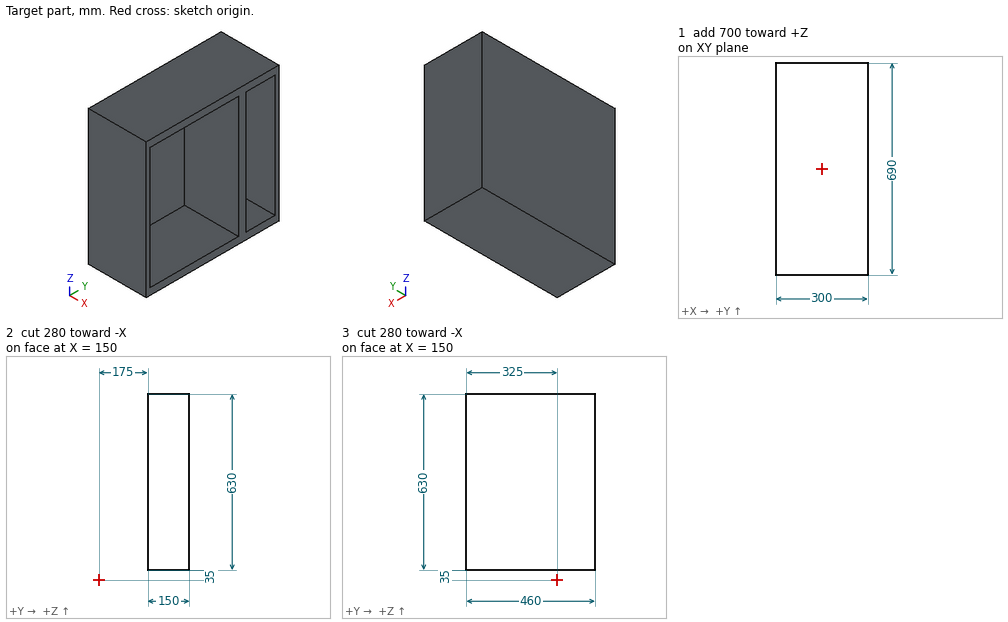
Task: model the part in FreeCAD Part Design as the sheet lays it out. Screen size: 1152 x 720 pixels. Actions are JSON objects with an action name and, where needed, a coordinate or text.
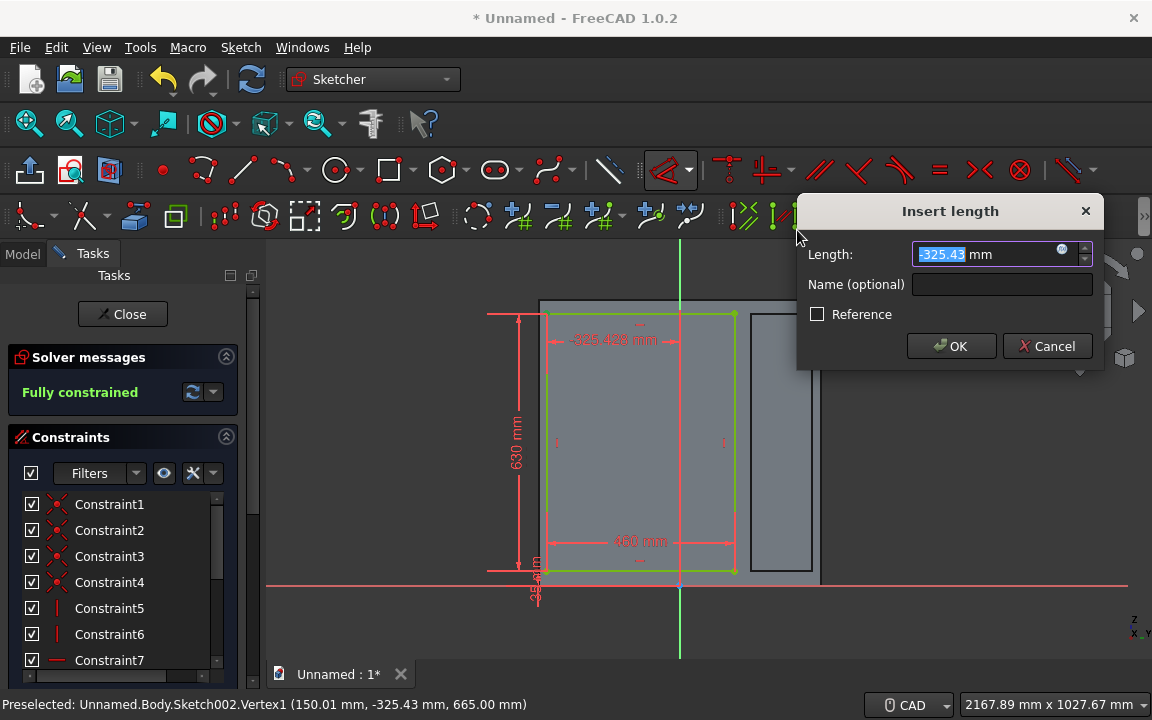
{"action": "type", "text": "-325"}
{"action": "key", "text": "Return"}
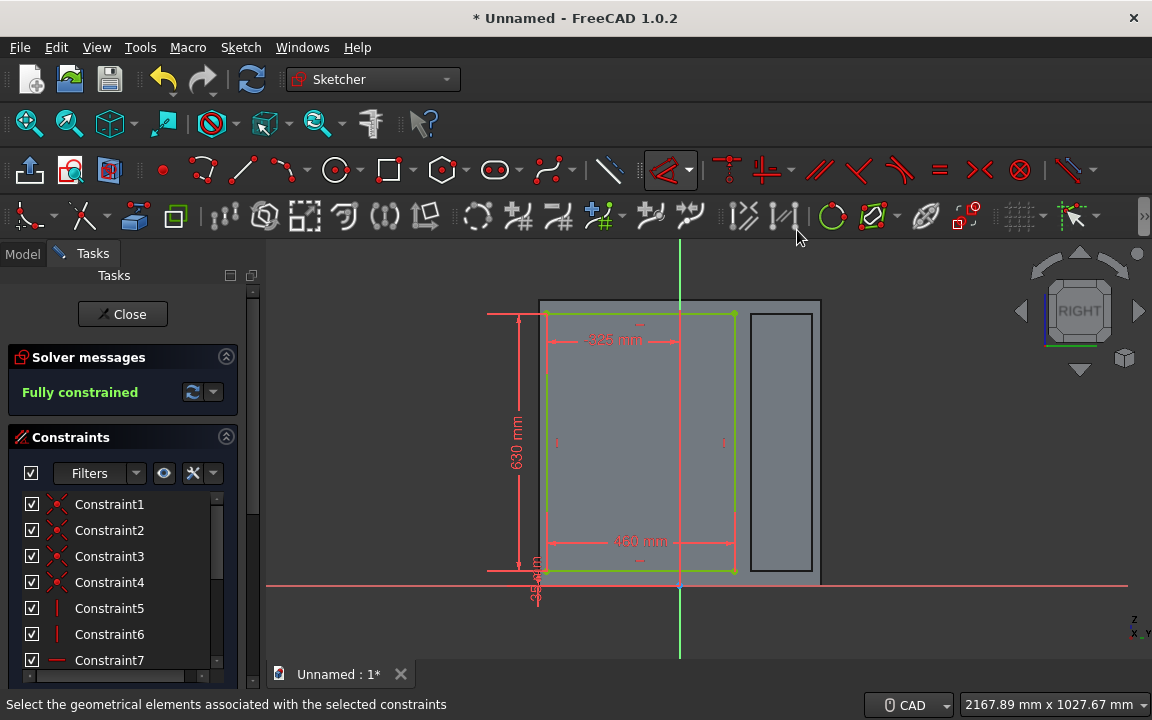
{"action": "left_click", "coordinate": [123, 314]}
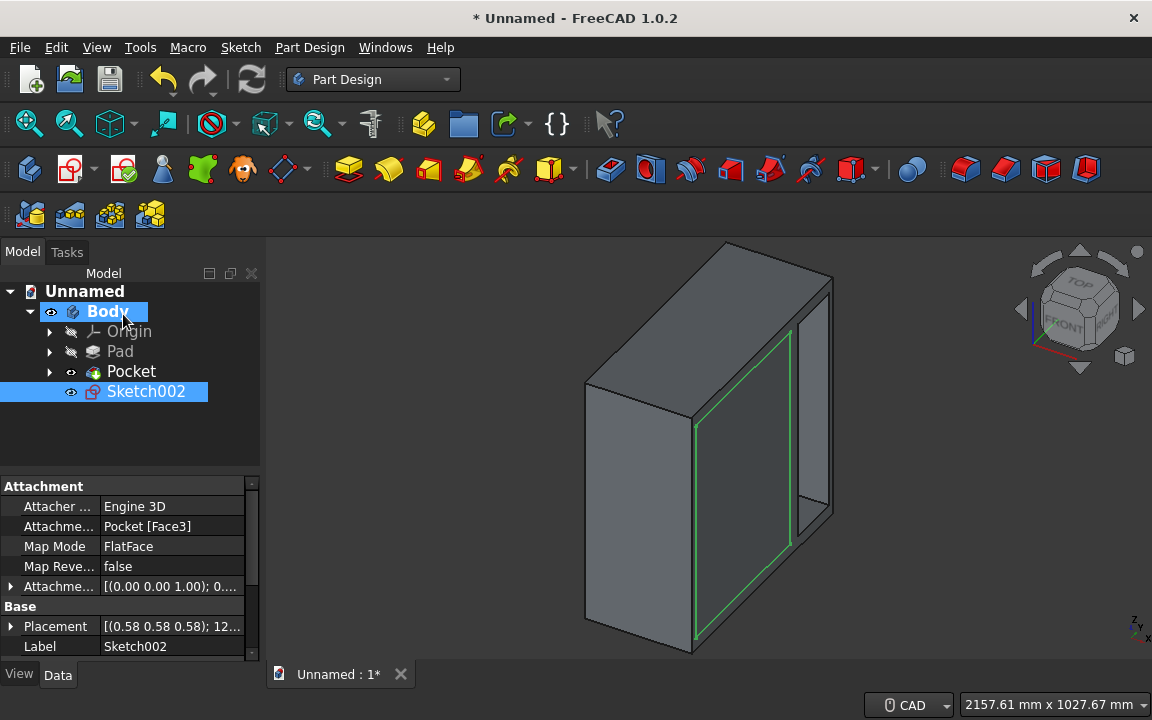
{"action": "left_click", "coordinate": [612, 170]}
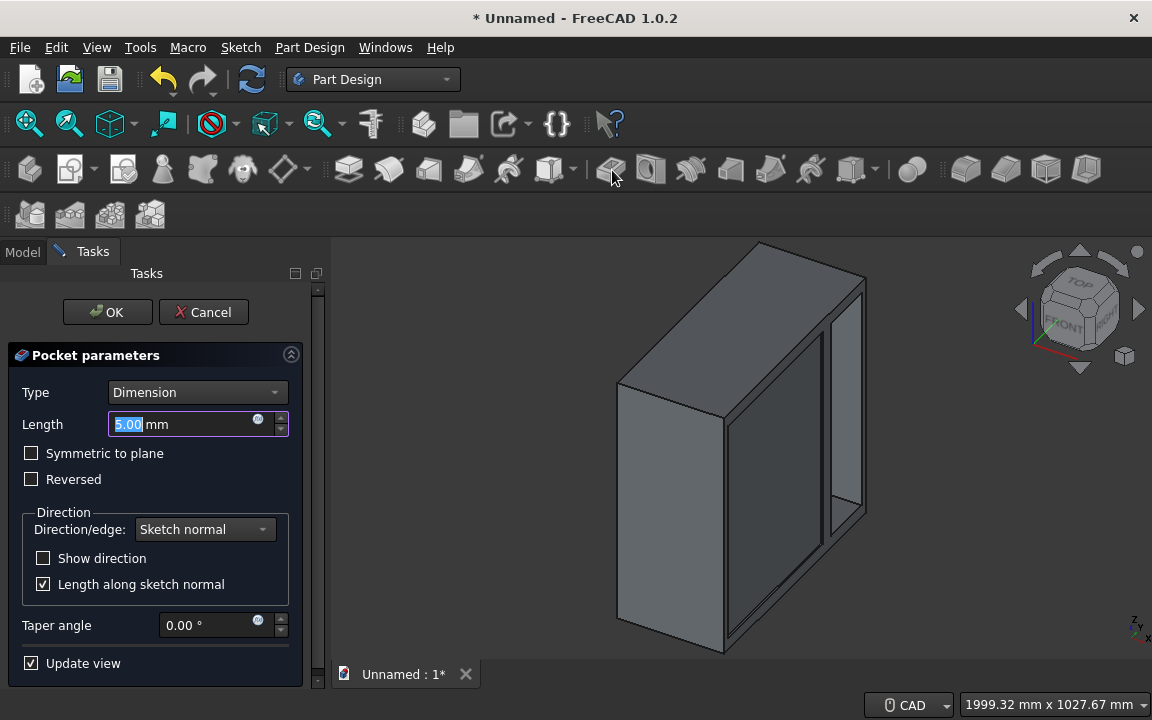
{"action": "type", "text": "280"}
{"action": "key", "text": "Tab"}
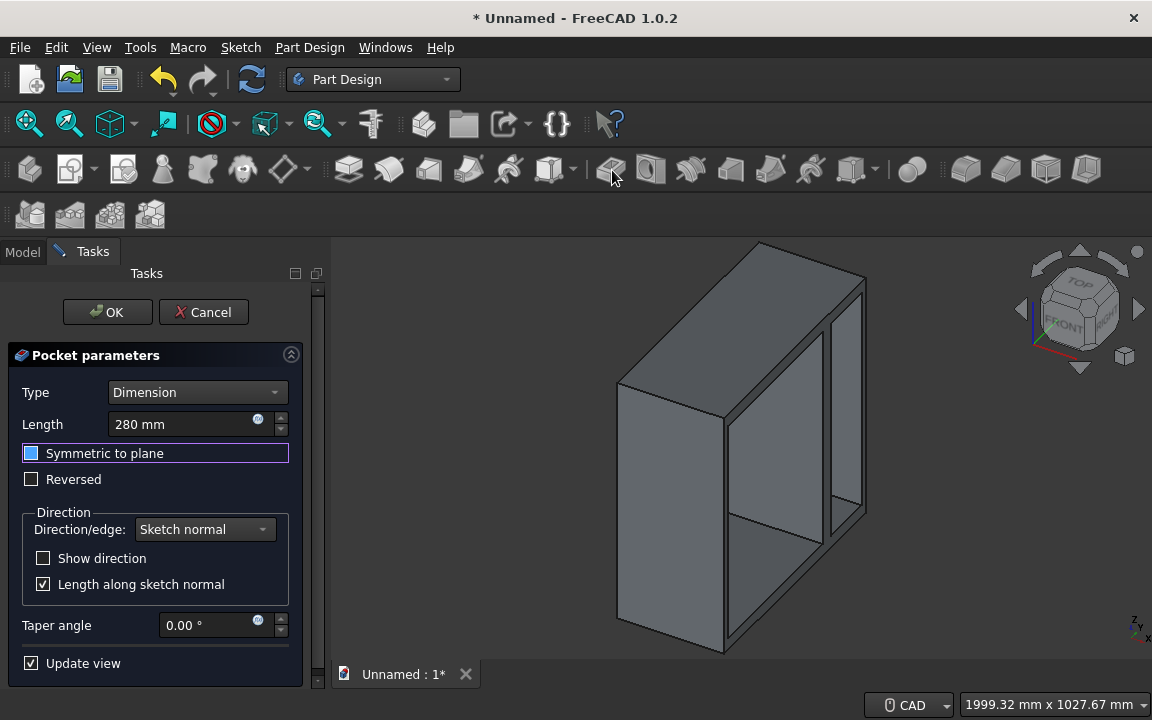
{"action": "left_click", "coordinate": [108, 312]}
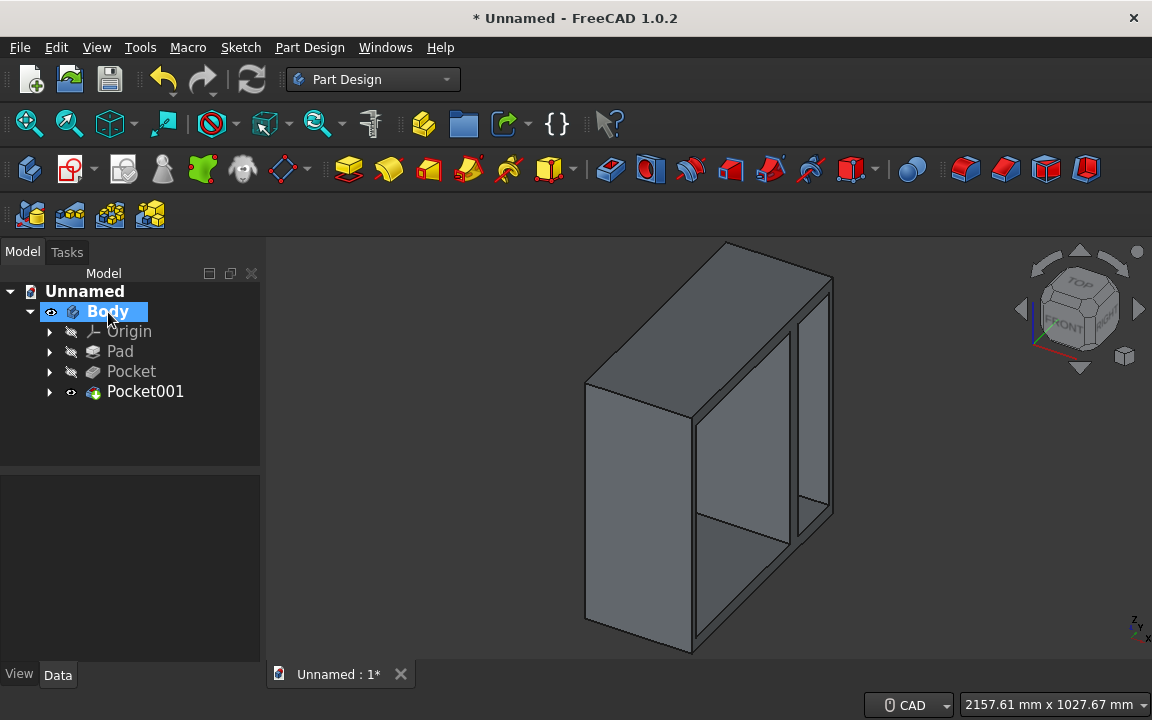
{"action": "key", "text": "0"}